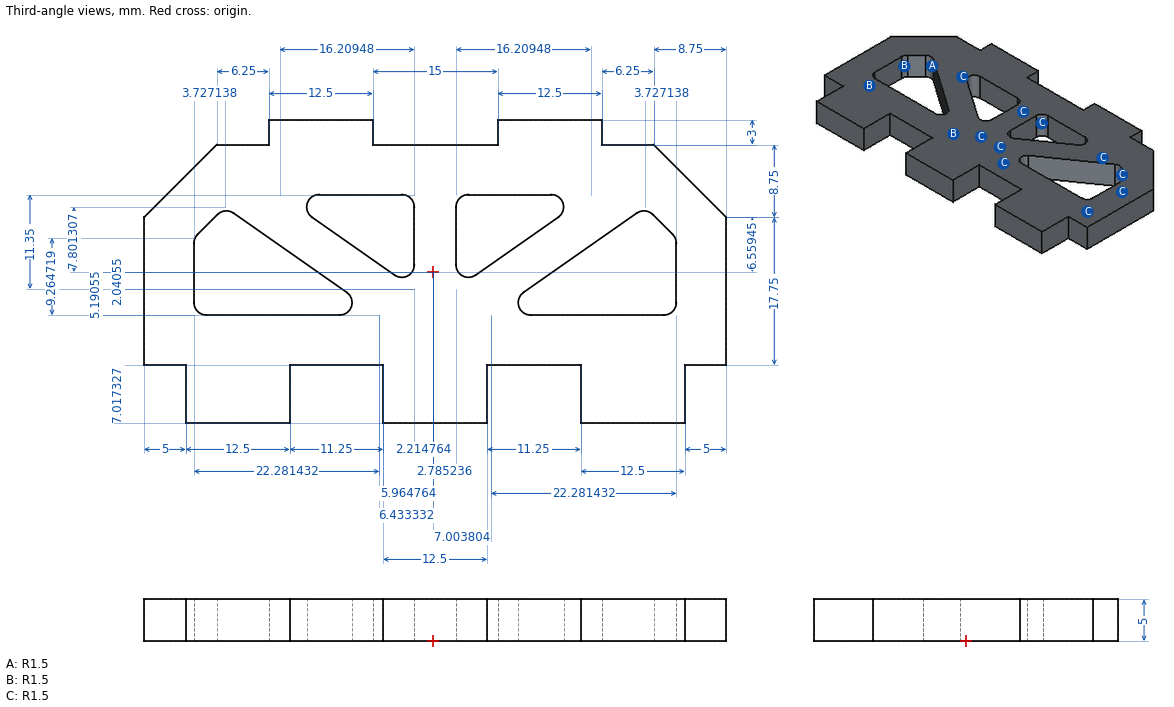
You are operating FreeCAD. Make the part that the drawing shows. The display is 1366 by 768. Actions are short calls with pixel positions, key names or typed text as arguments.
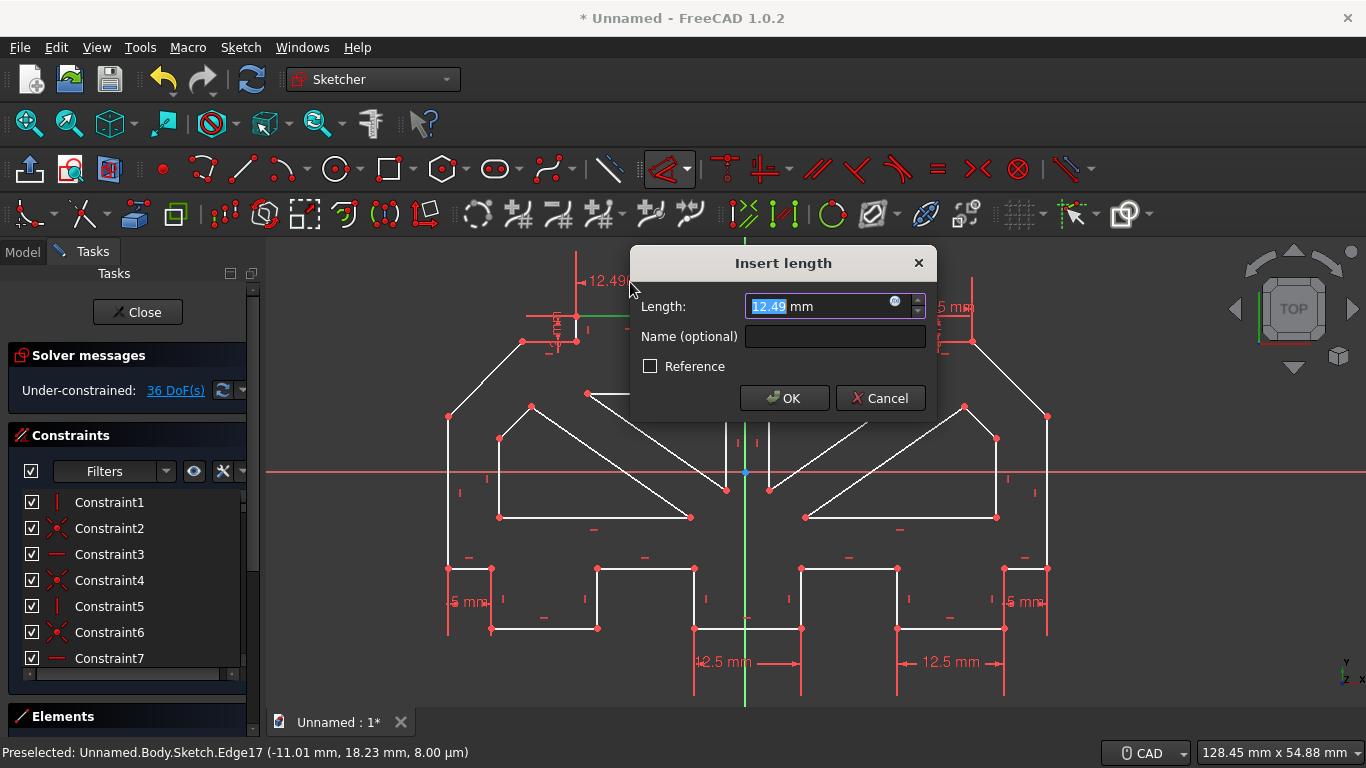
text(12.5)
key(Return)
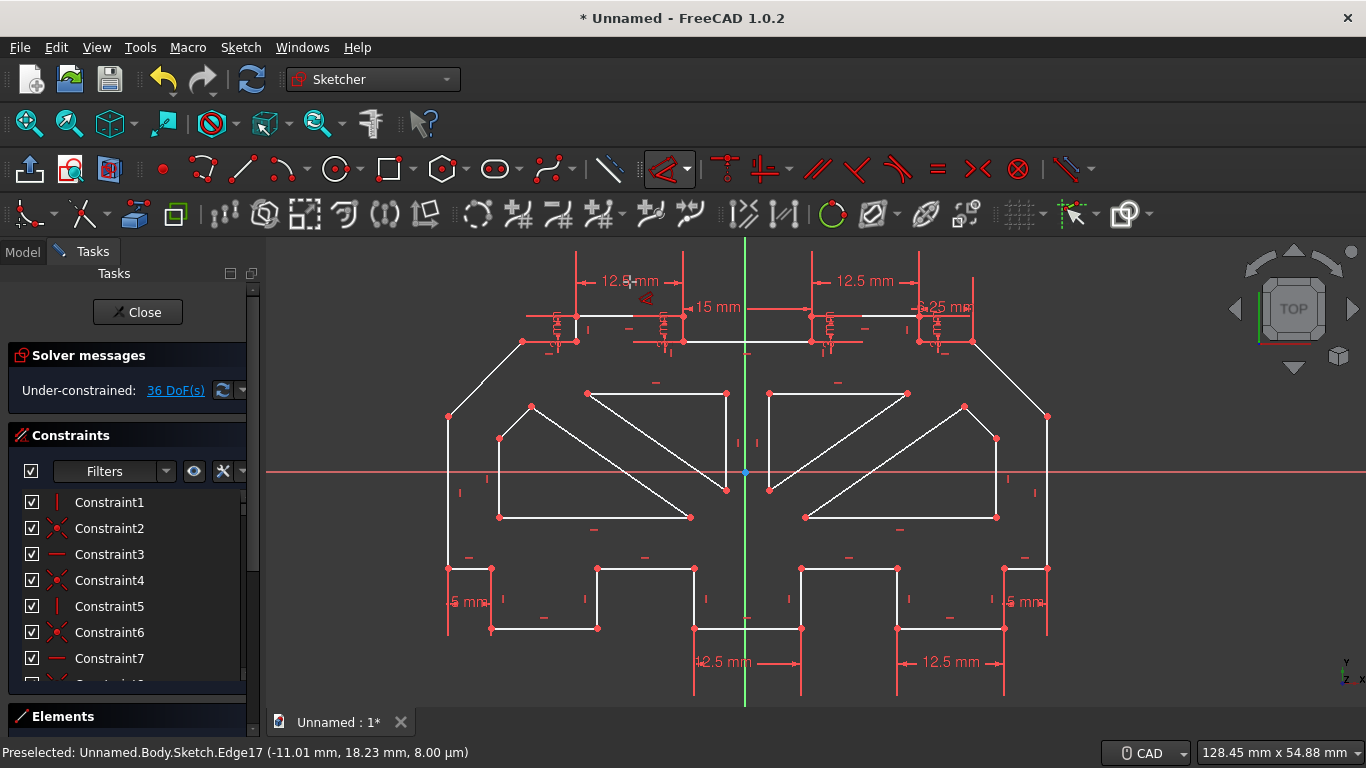
click(560, 342)
click(549, 308)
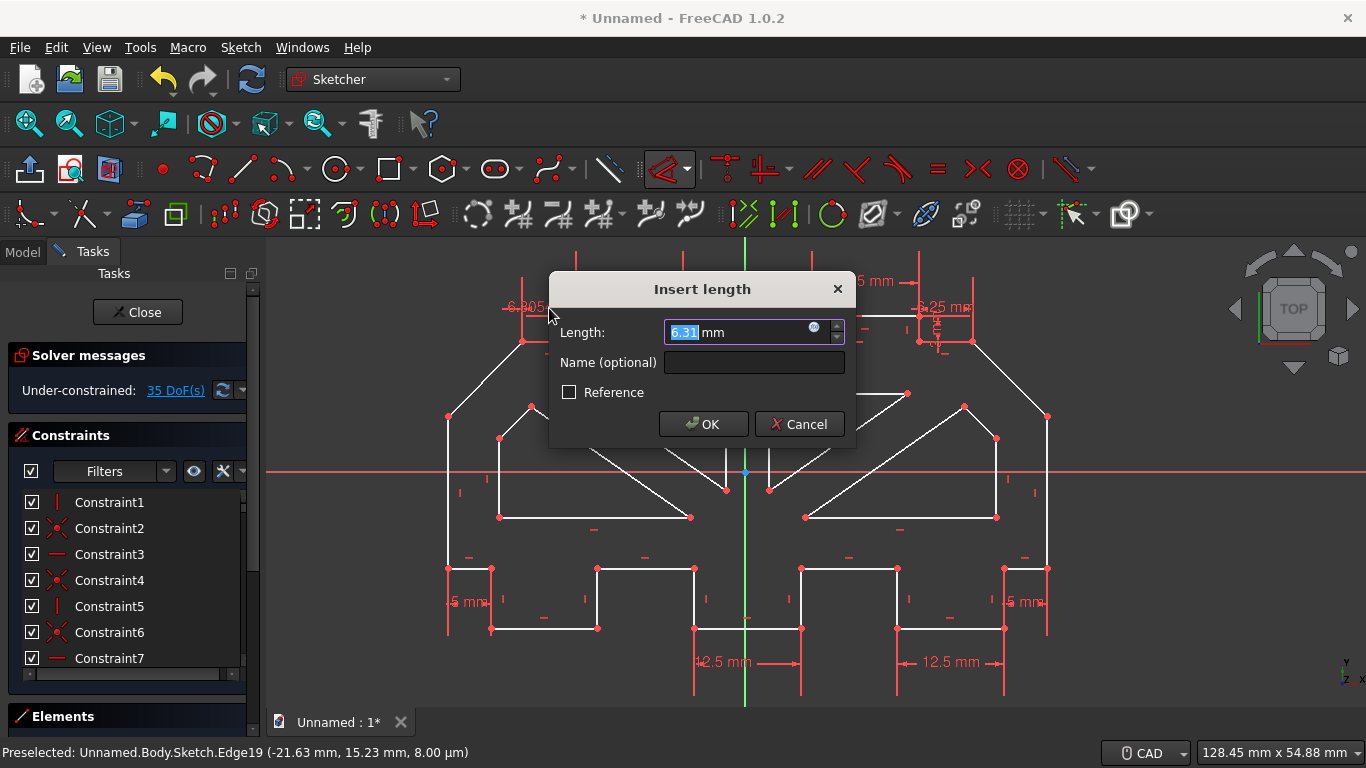
text(6.25)
key(Return)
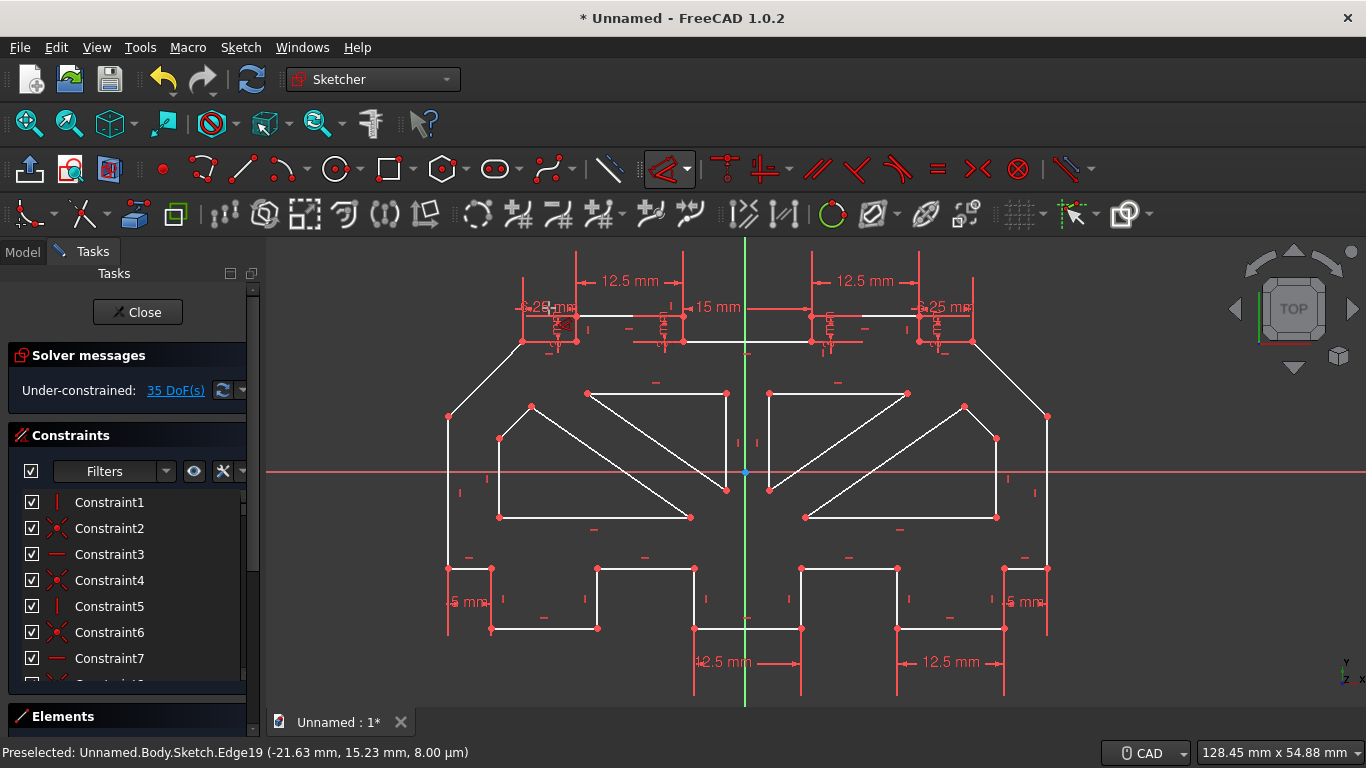
click(523, 629)
click(544, 663)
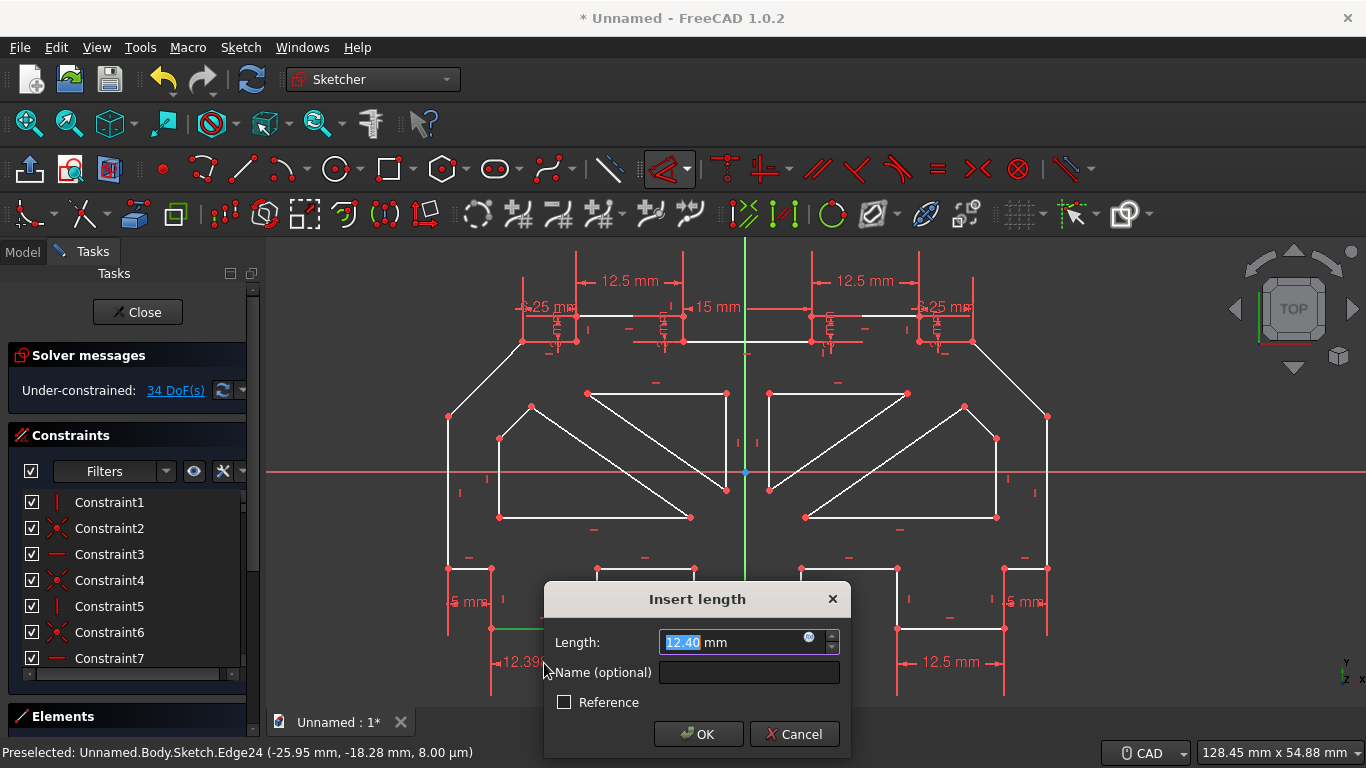
text(12.5)
key(Return)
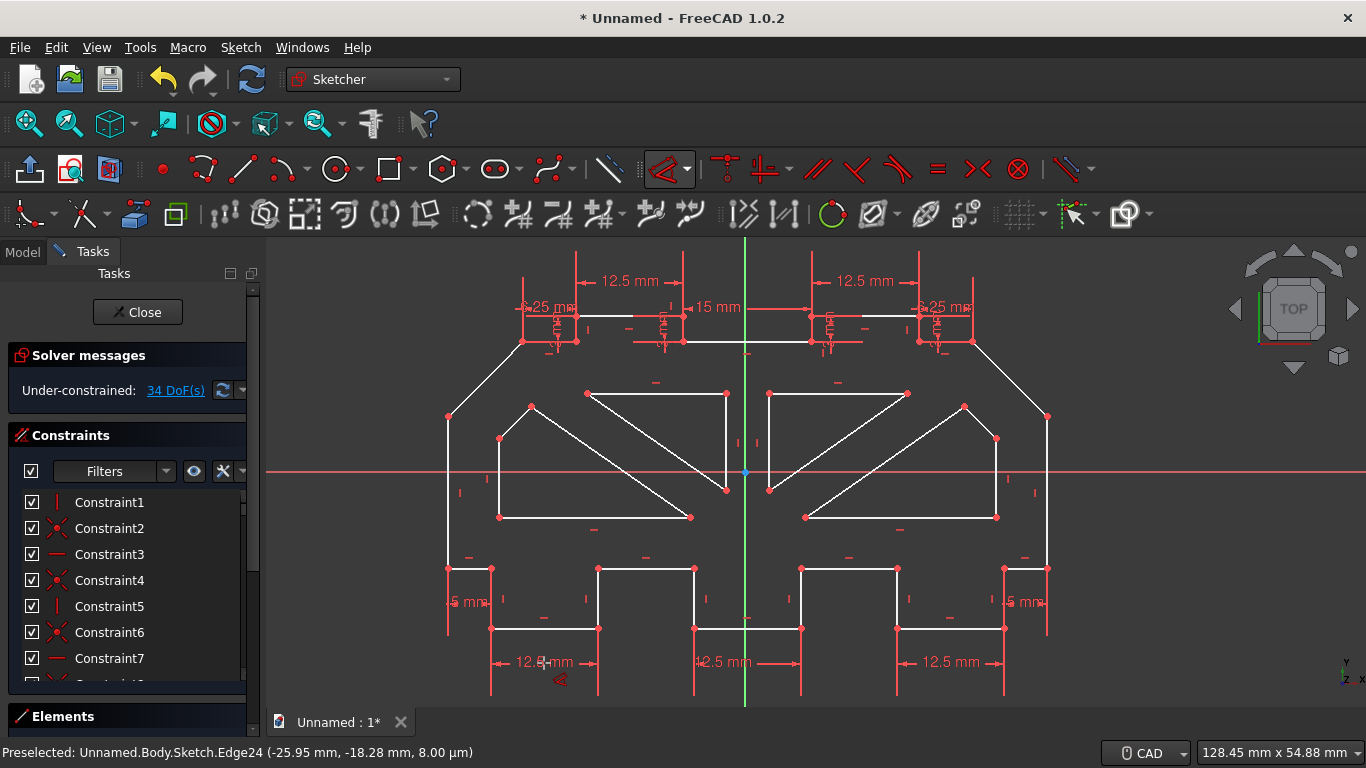
click(830, 569)
click(849, 603)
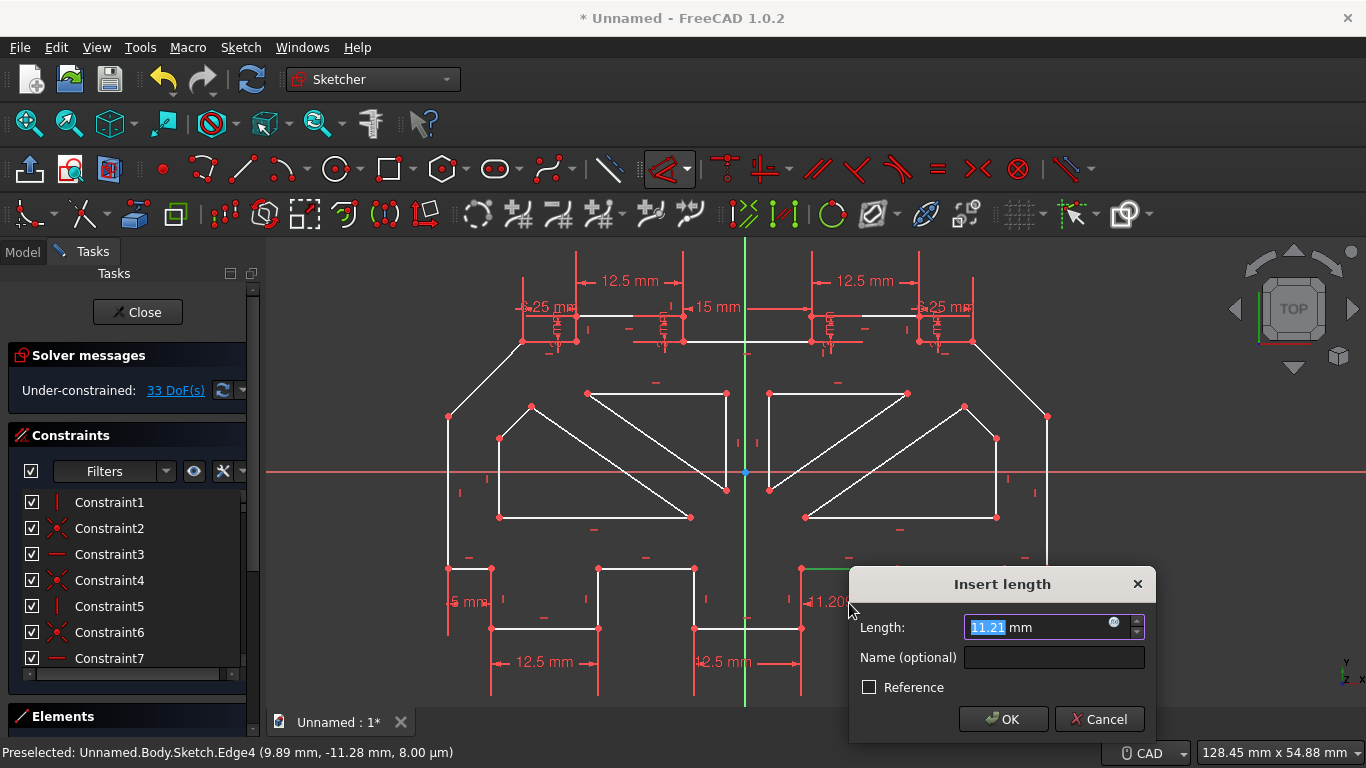
text(11.25)
key(Return)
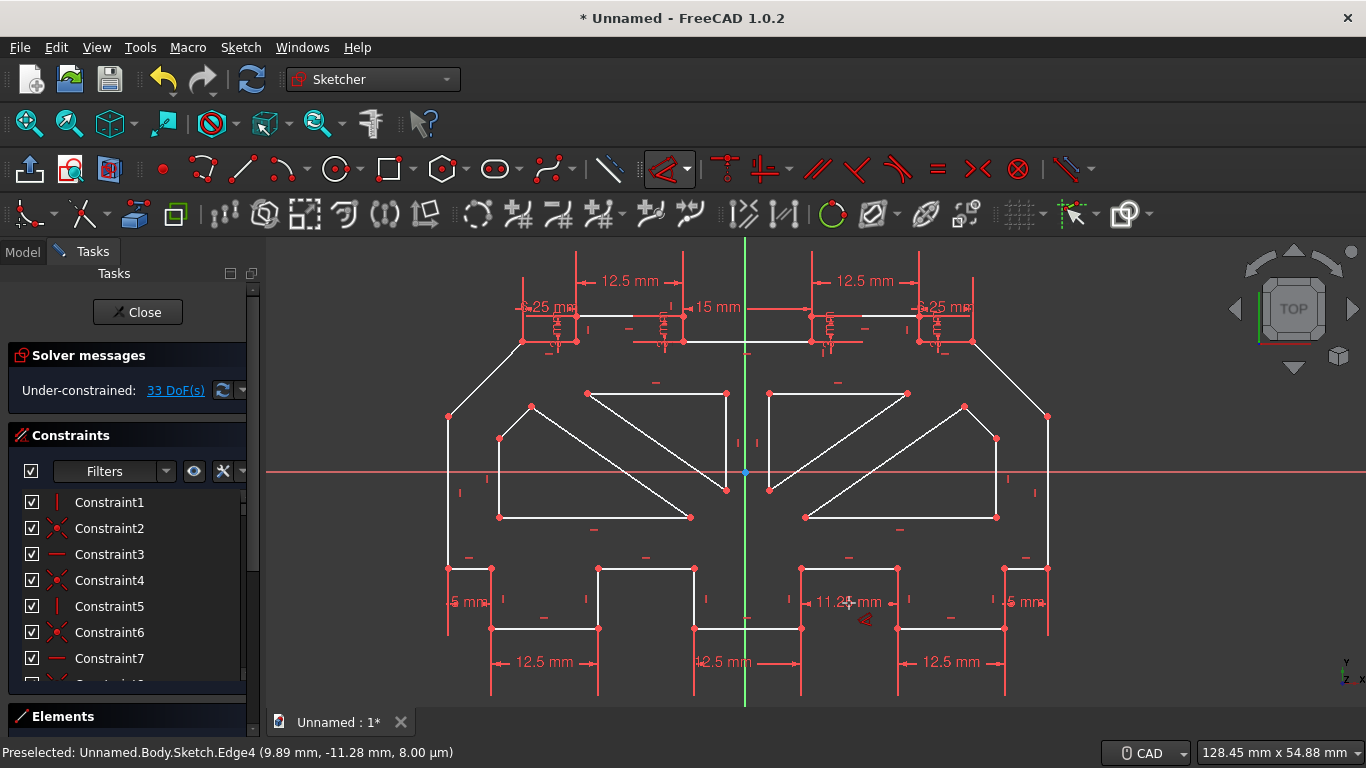
click(1048, 523)
click(1082, 493)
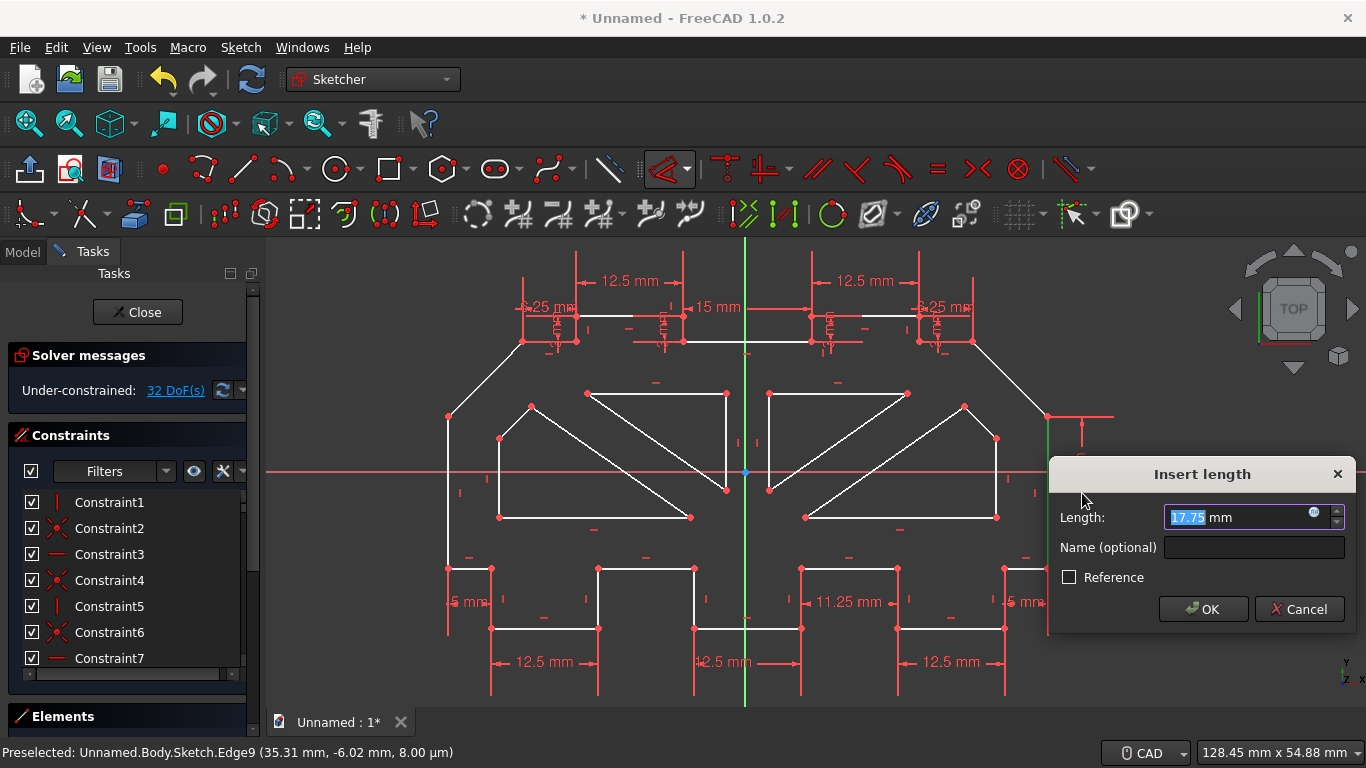
text(17.75)
key(Return)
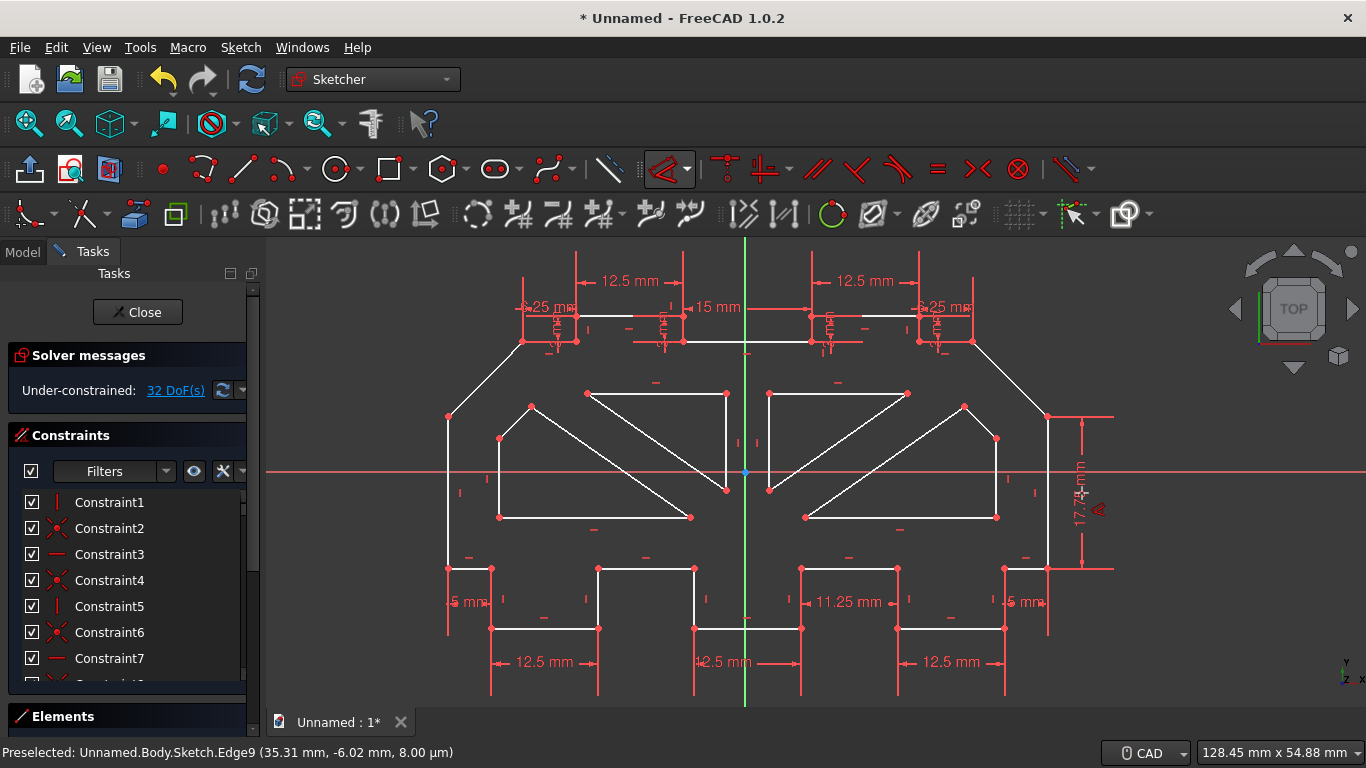
scroll(448, 463, up, 2)